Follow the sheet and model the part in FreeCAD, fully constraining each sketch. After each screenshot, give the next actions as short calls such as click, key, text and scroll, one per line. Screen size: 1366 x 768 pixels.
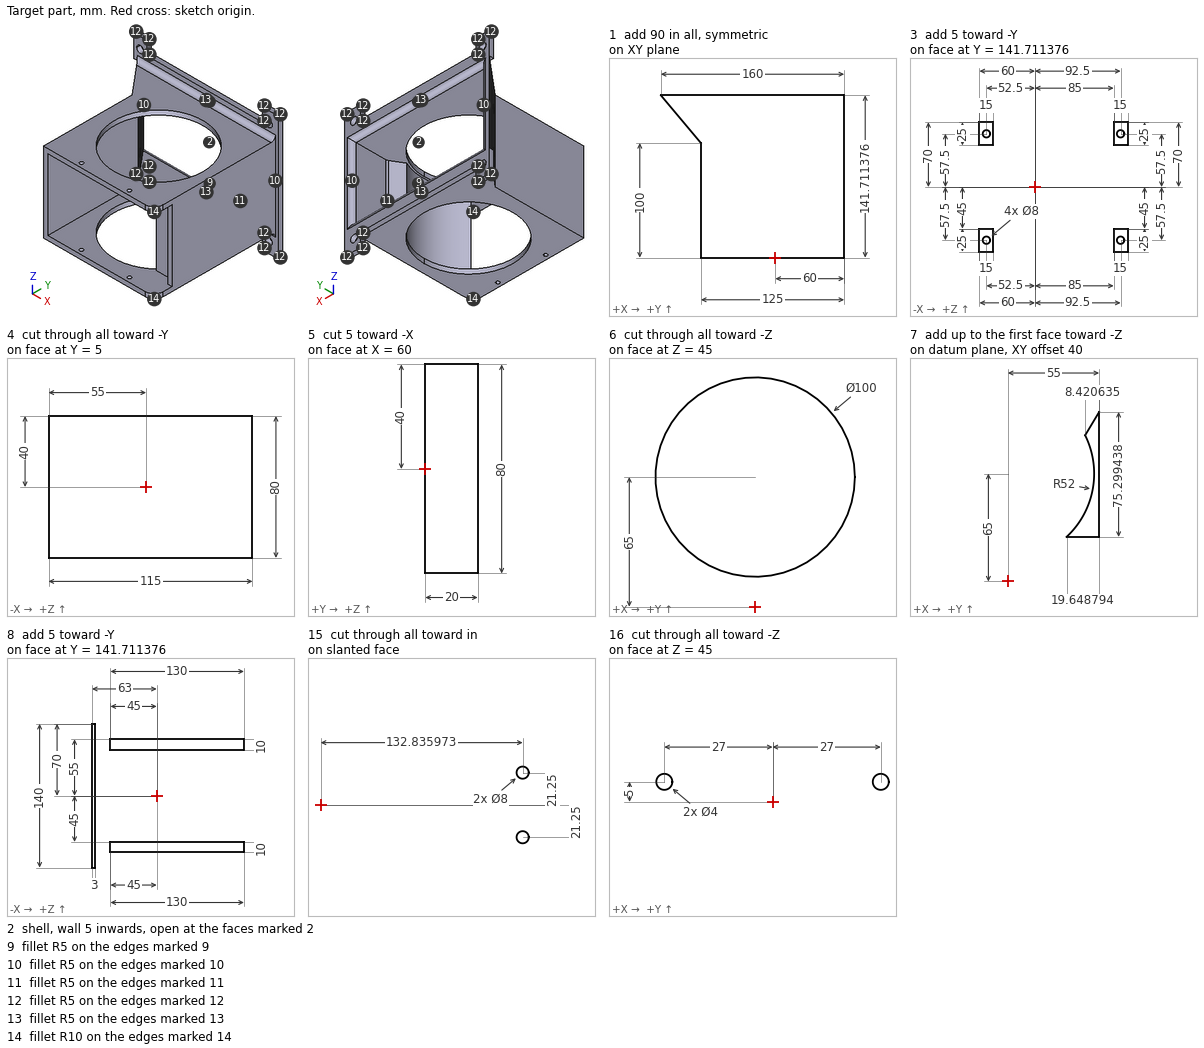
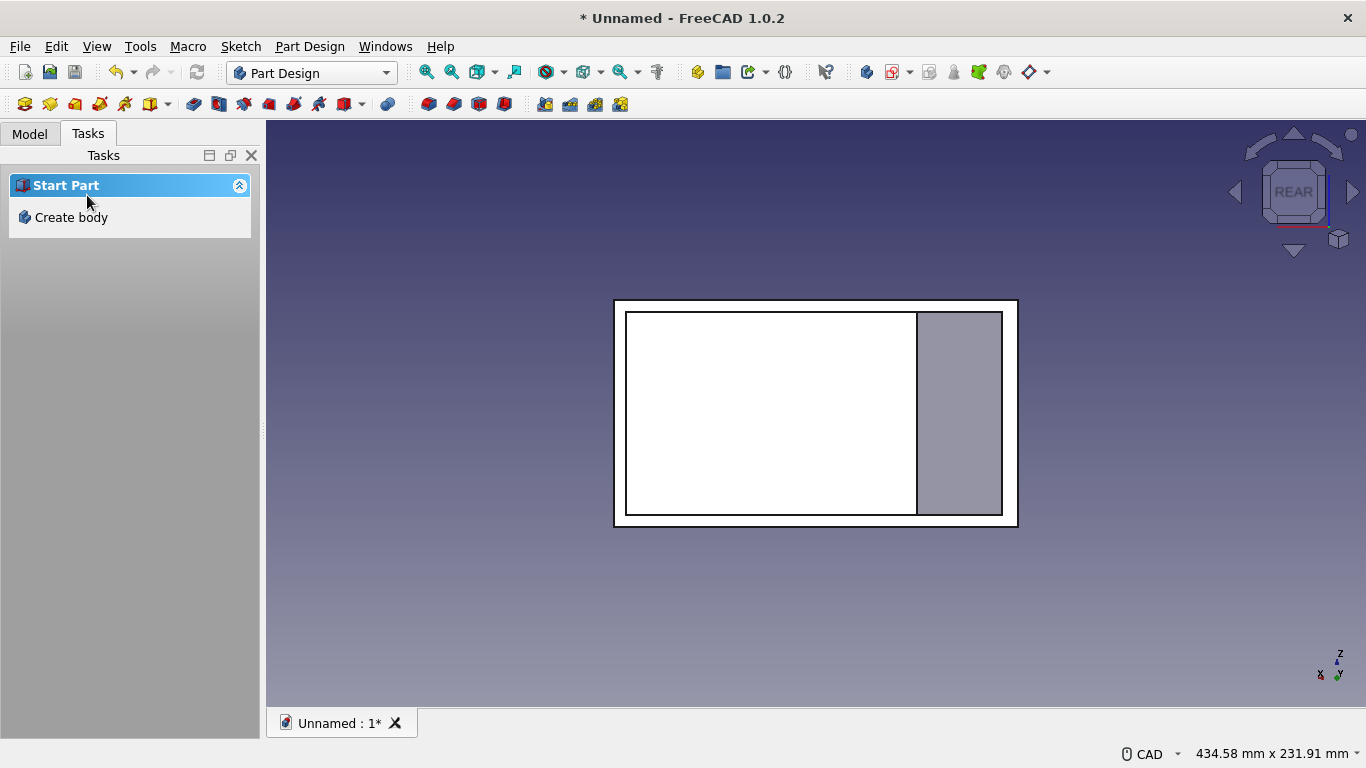
key(v)
key(f)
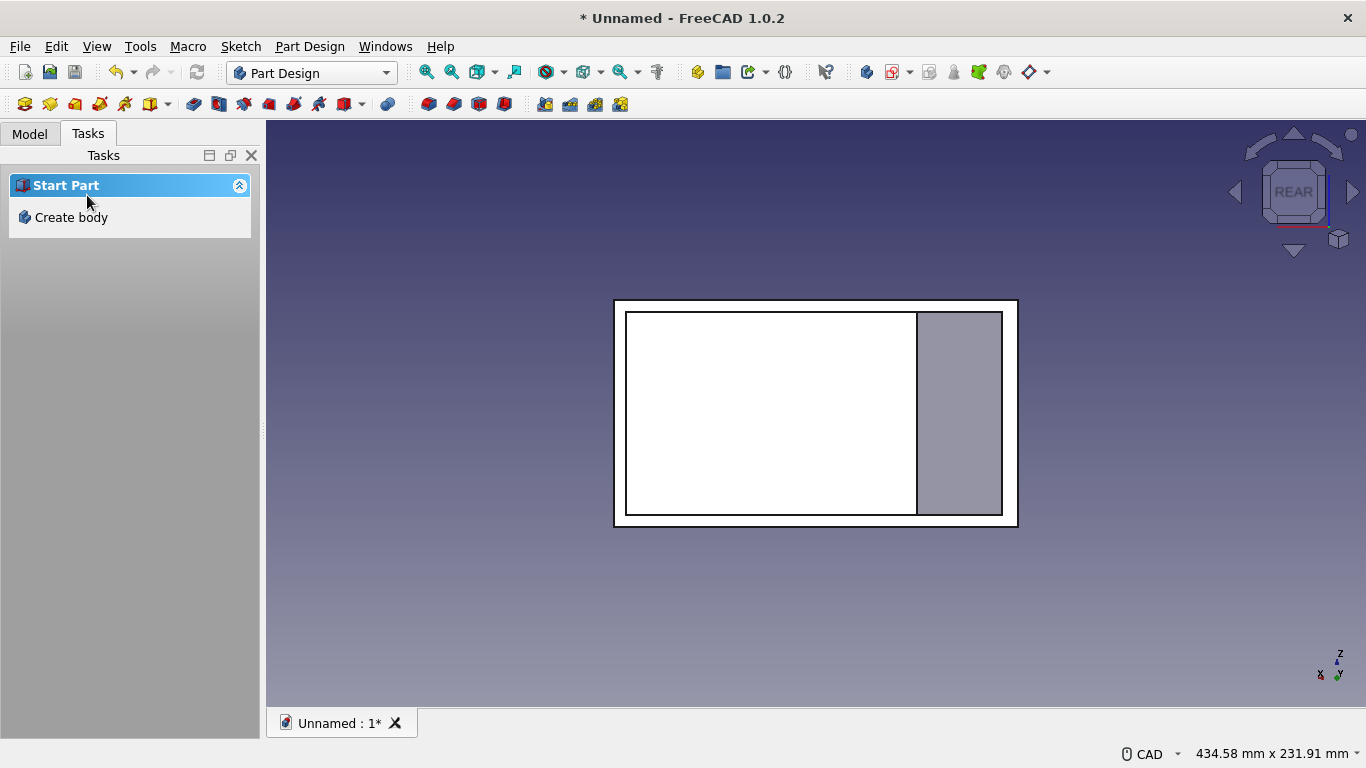
scroll(1013, 446, up, 4)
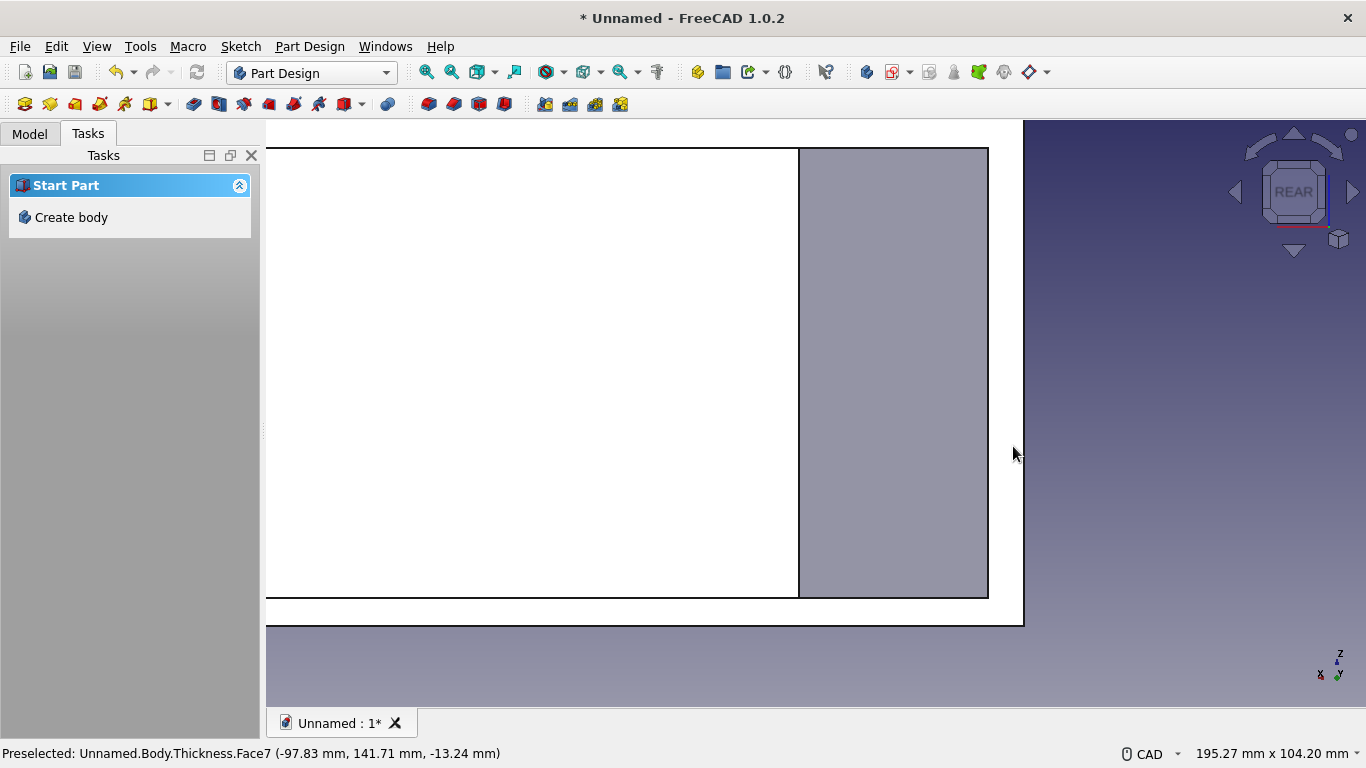
click(1012, 447)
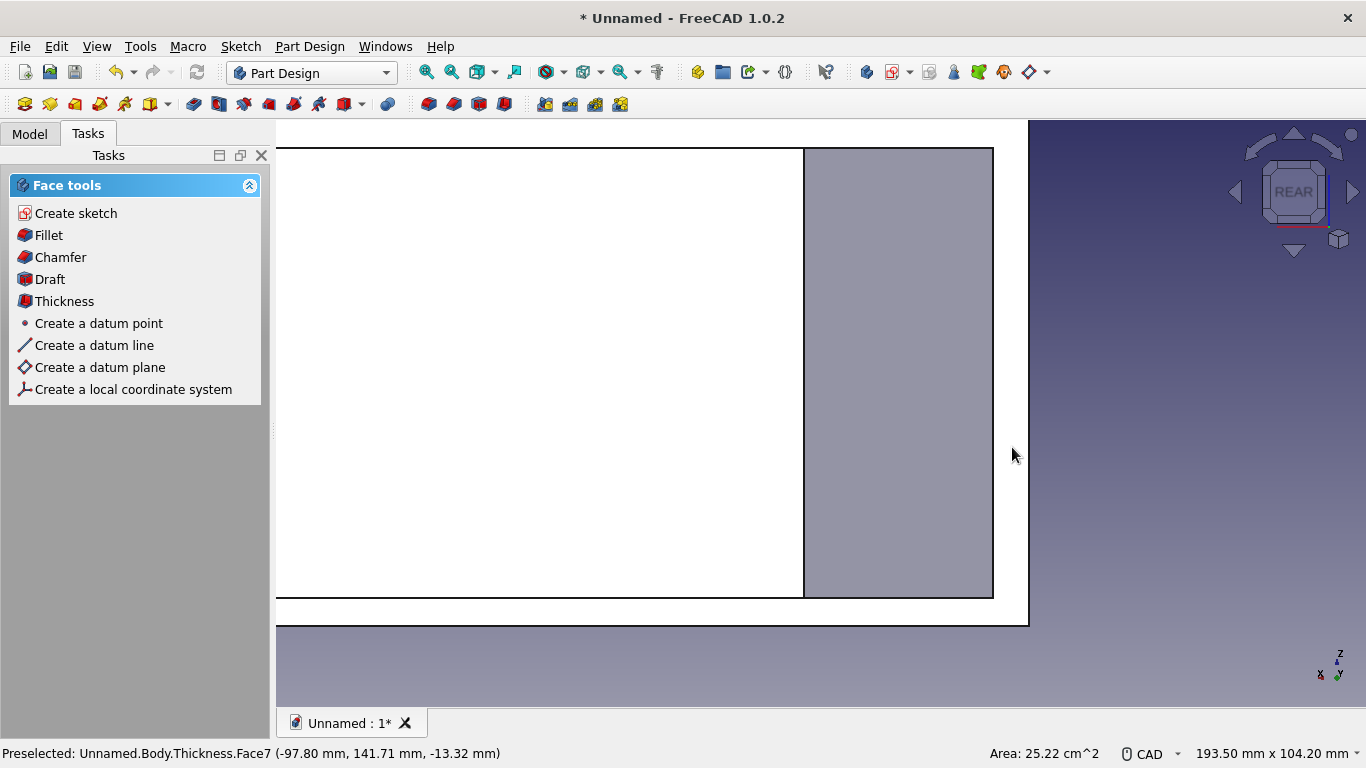
click(892, 72)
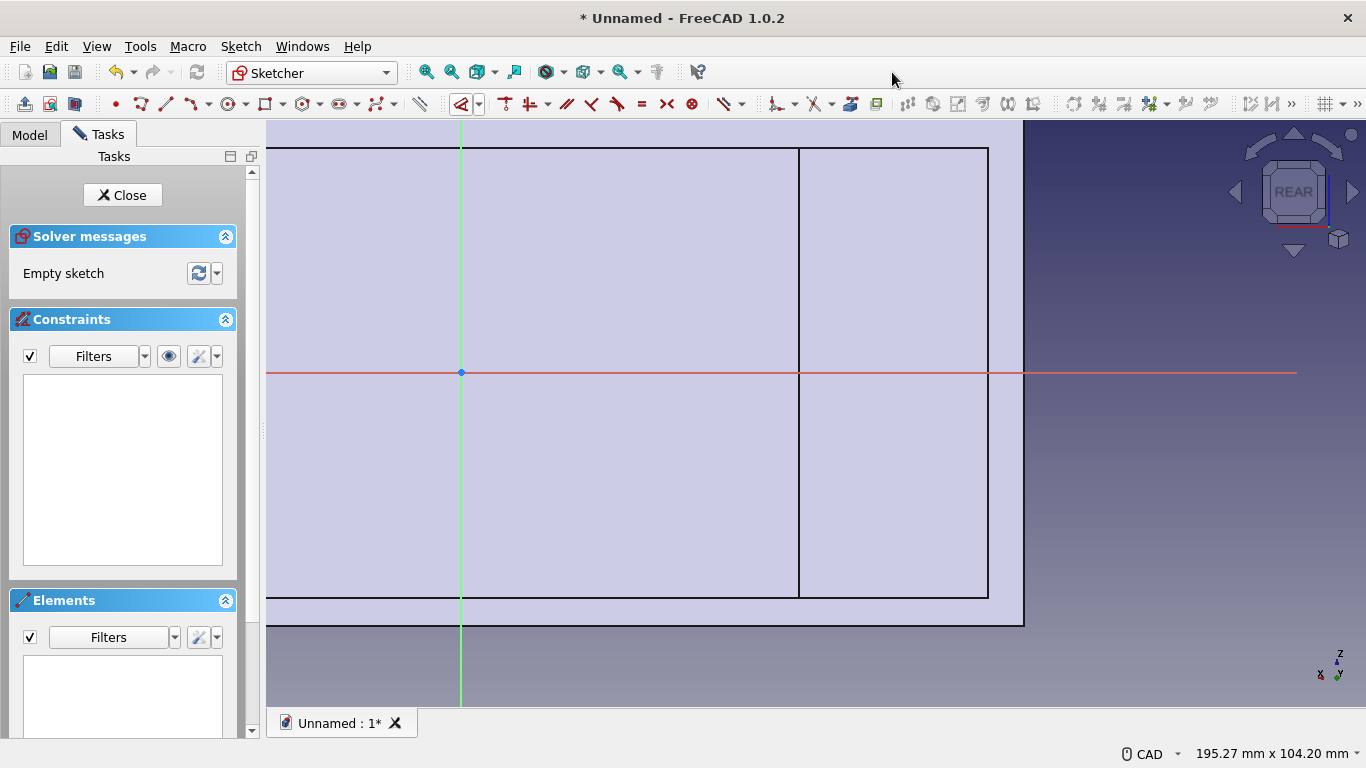
scroll(889, 447, down, 4)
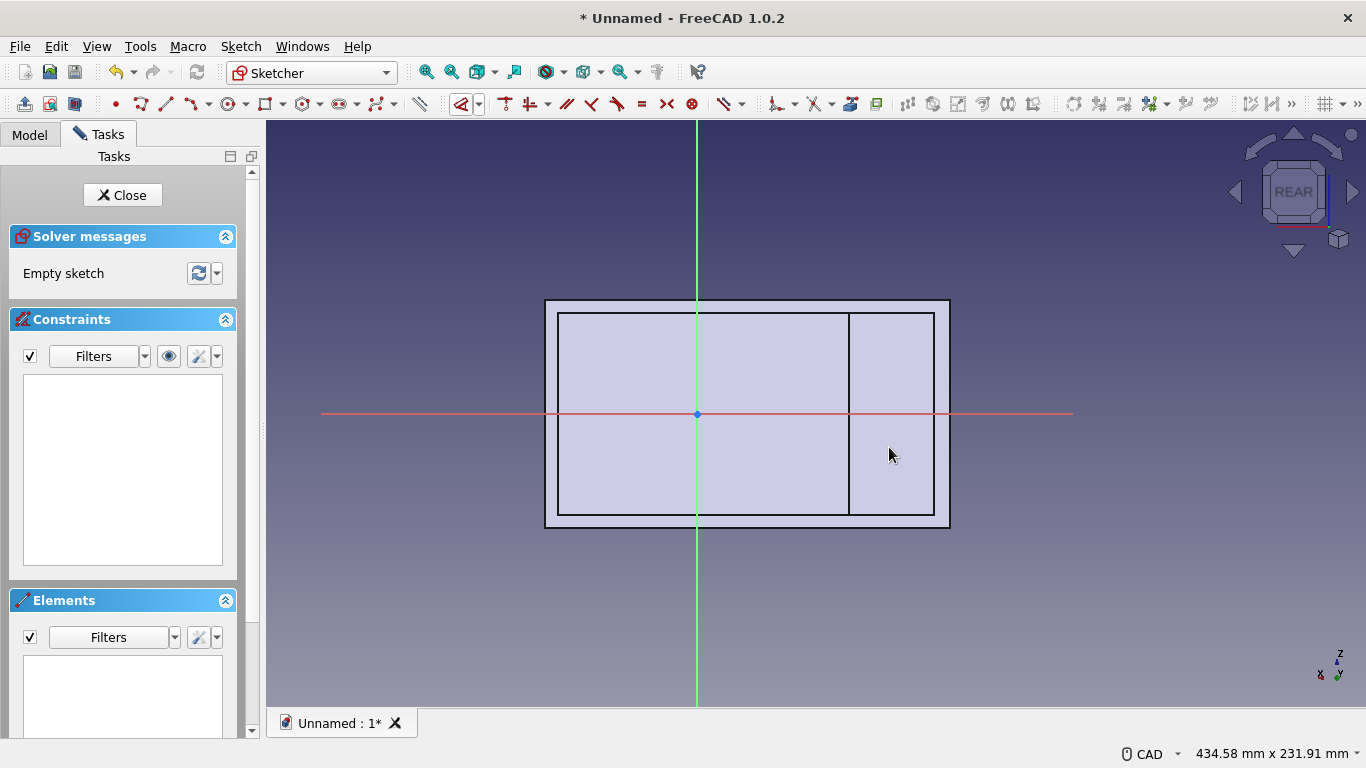
key(g)
key(r)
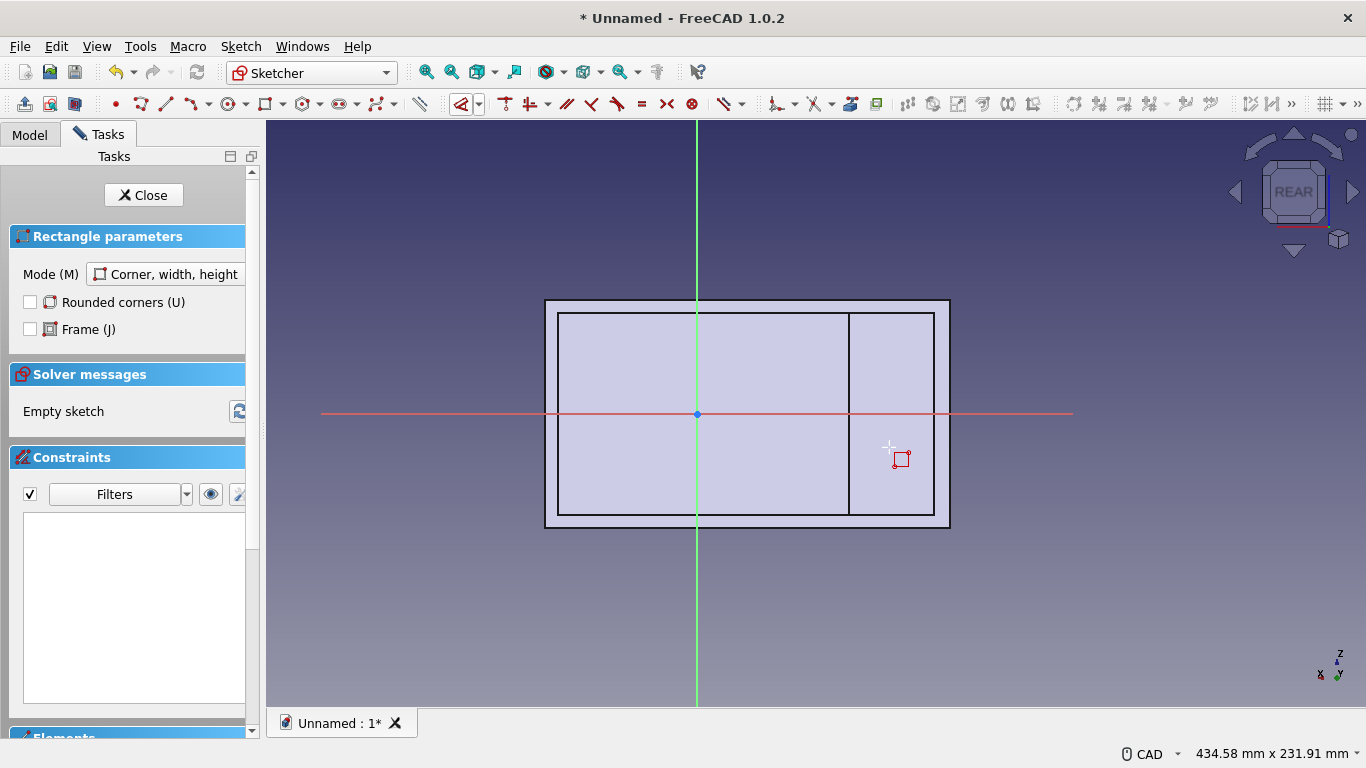
click(545, 528)
move(583, 591)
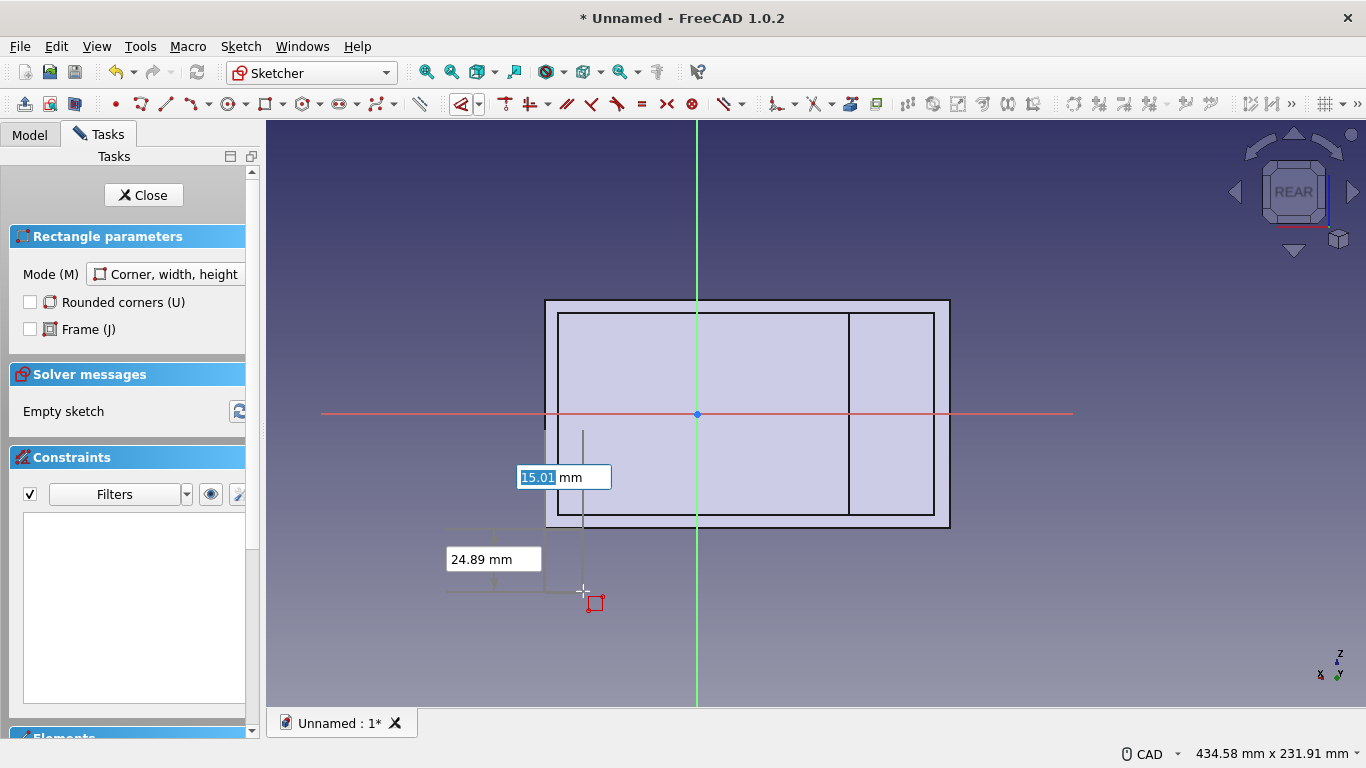
text(15)
key(Tab)
text(25)
key(Return)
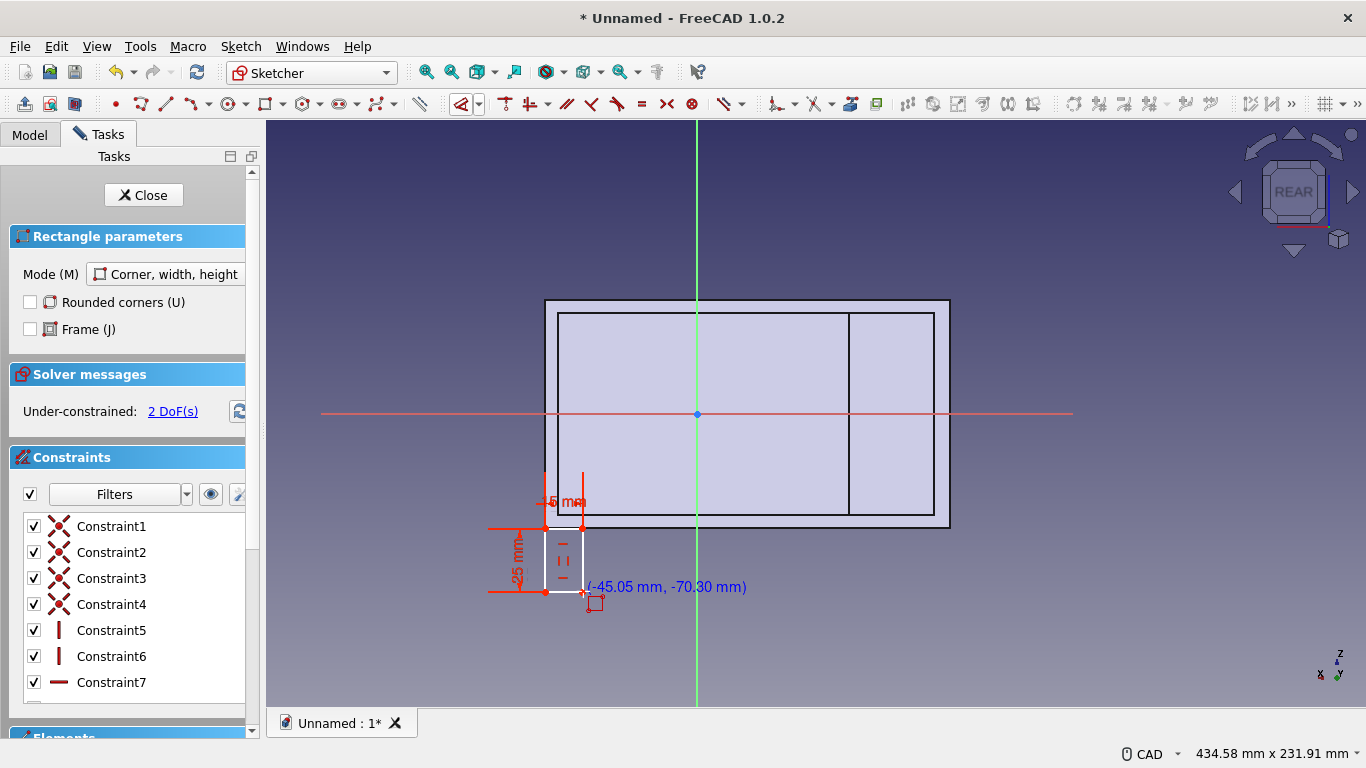
click(912, 237)
move(950, 300)